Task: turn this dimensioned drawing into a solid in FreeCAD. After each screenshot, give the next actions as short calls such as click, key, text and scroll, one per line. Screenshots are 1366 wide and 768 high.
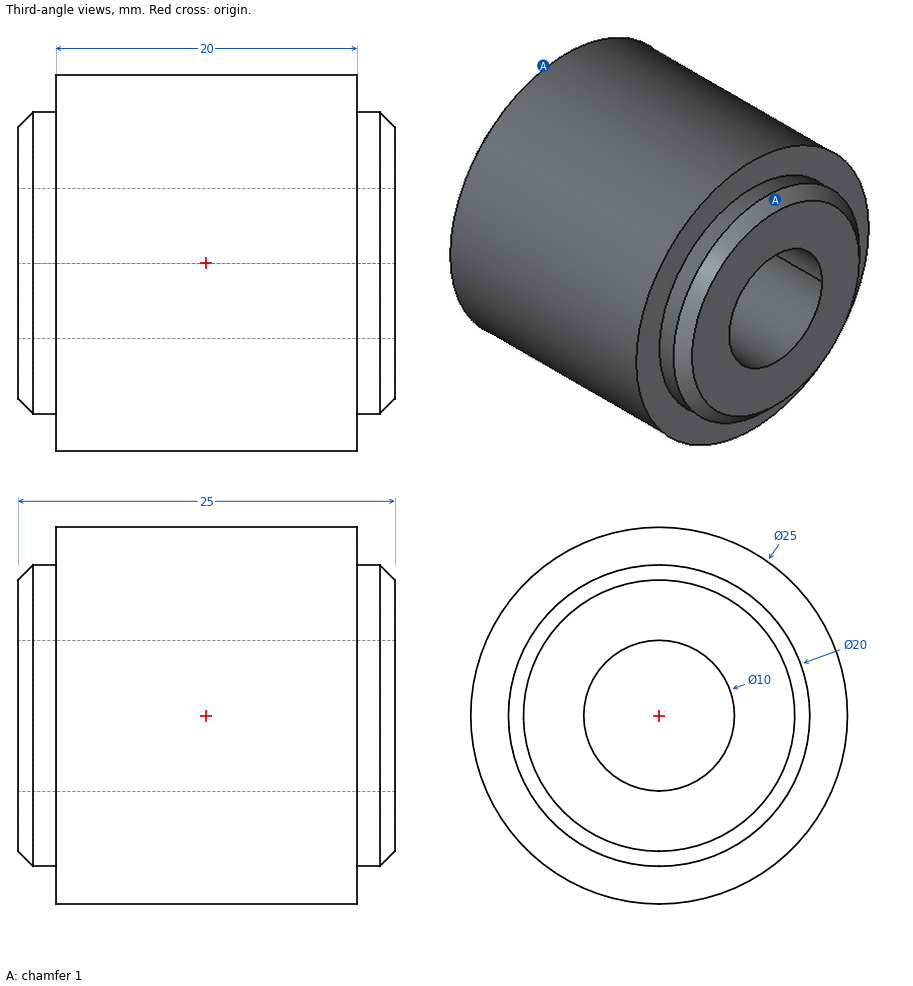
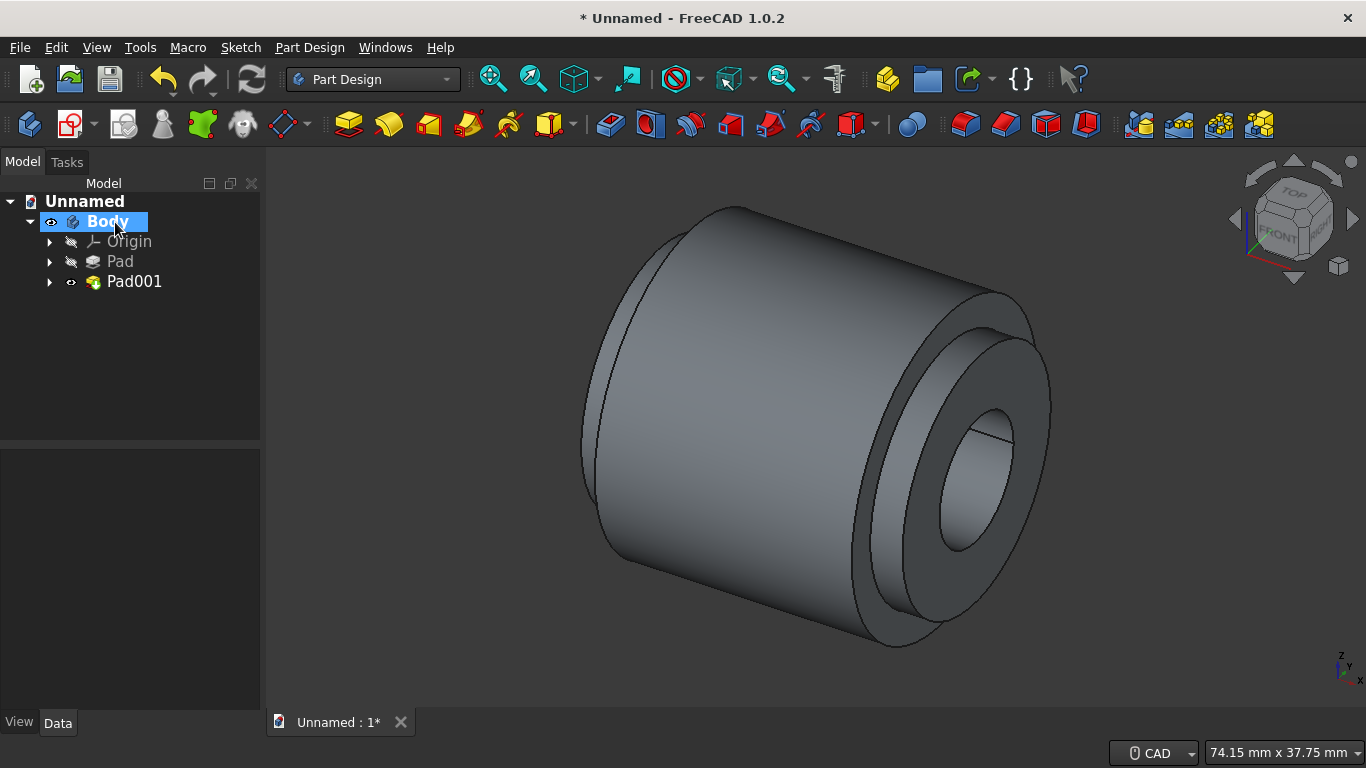
key(v)
key(f)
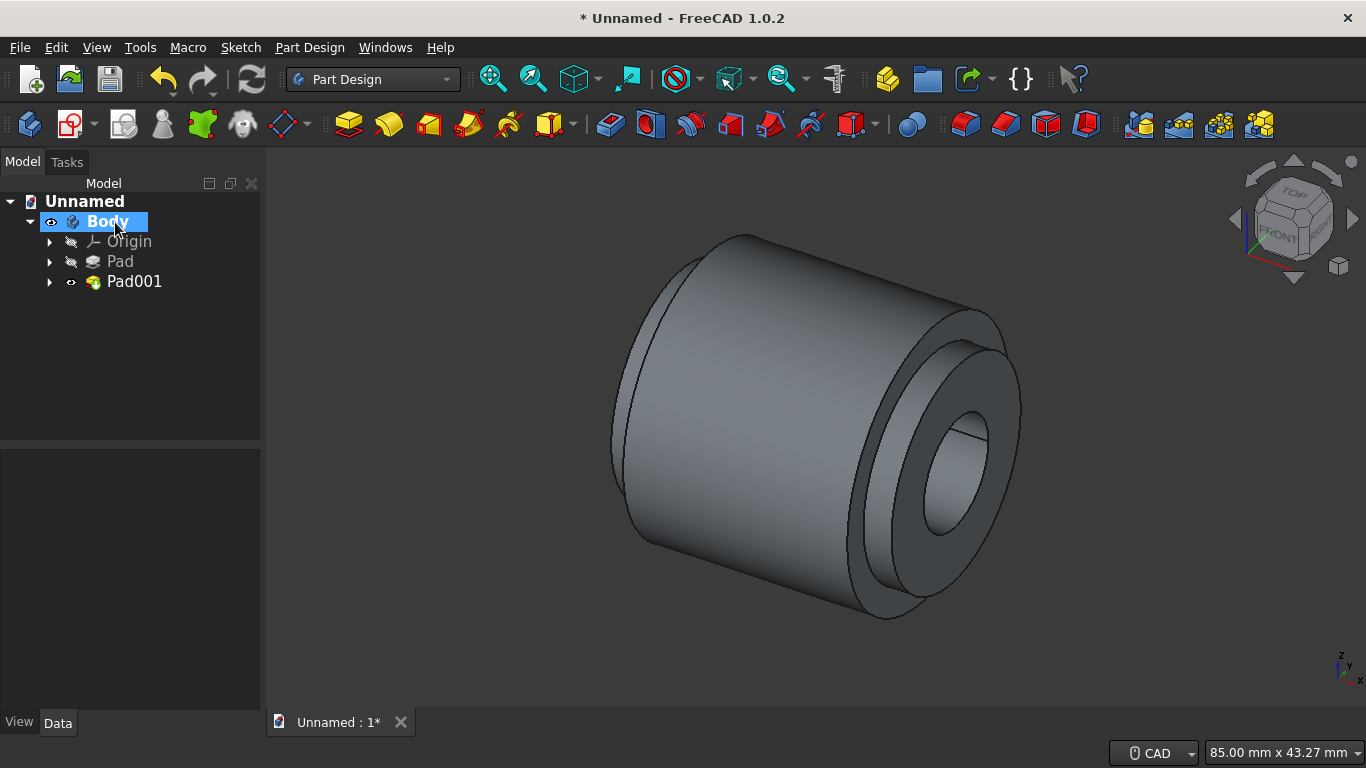
click(891, 537)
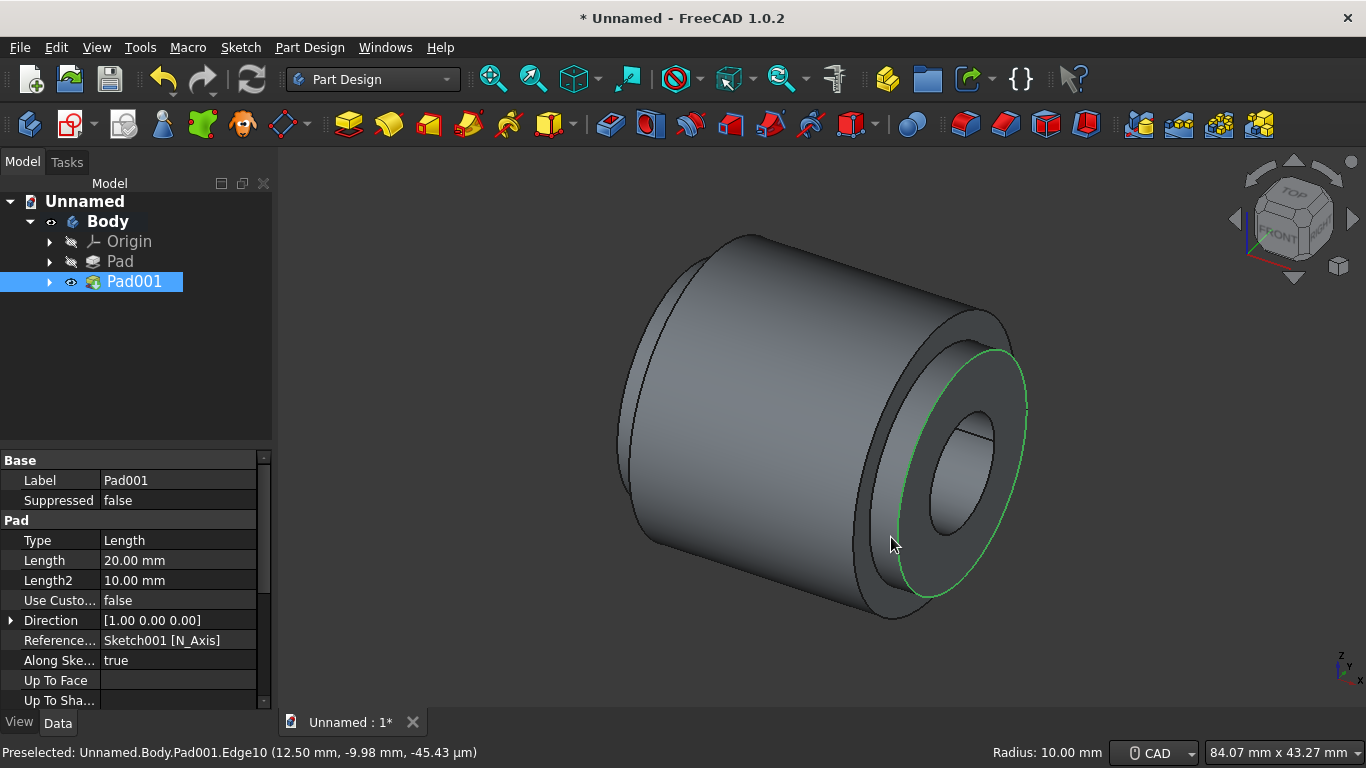
key(0)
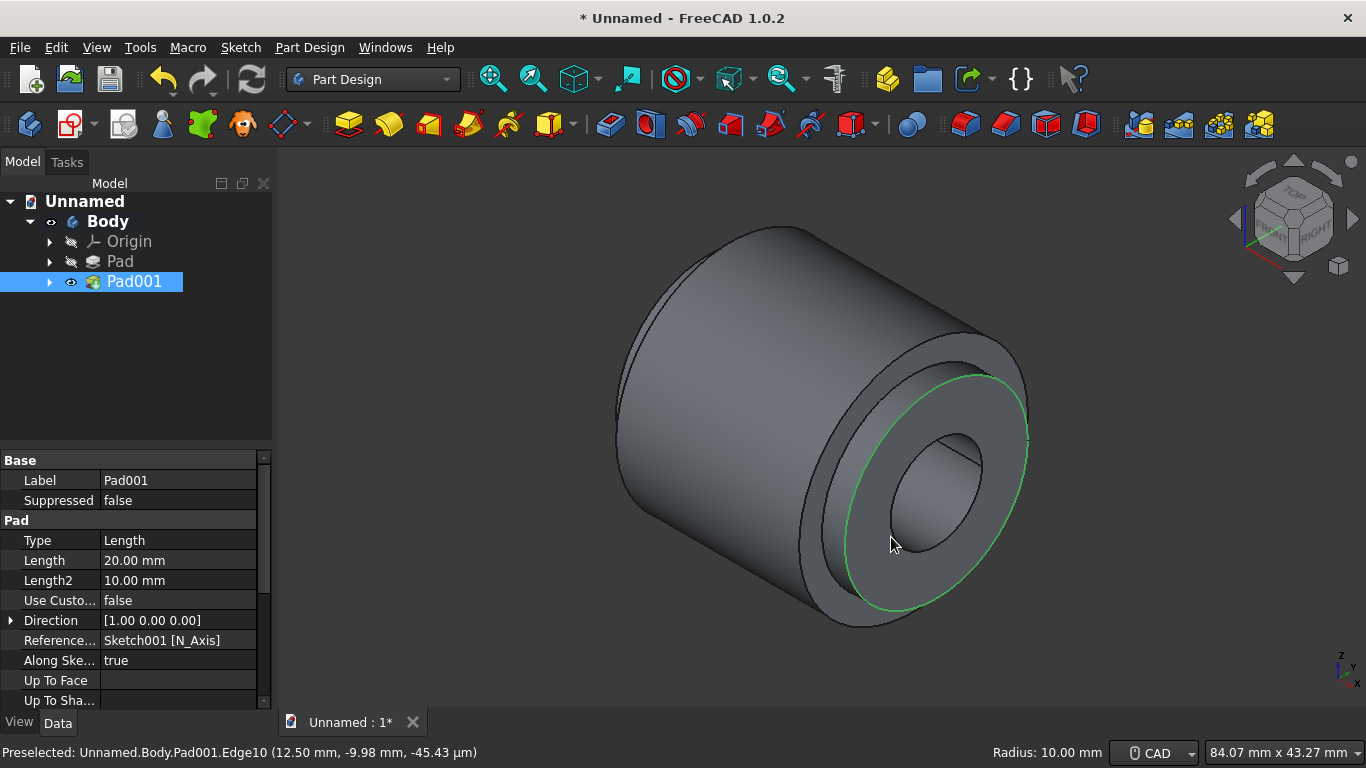
key(2)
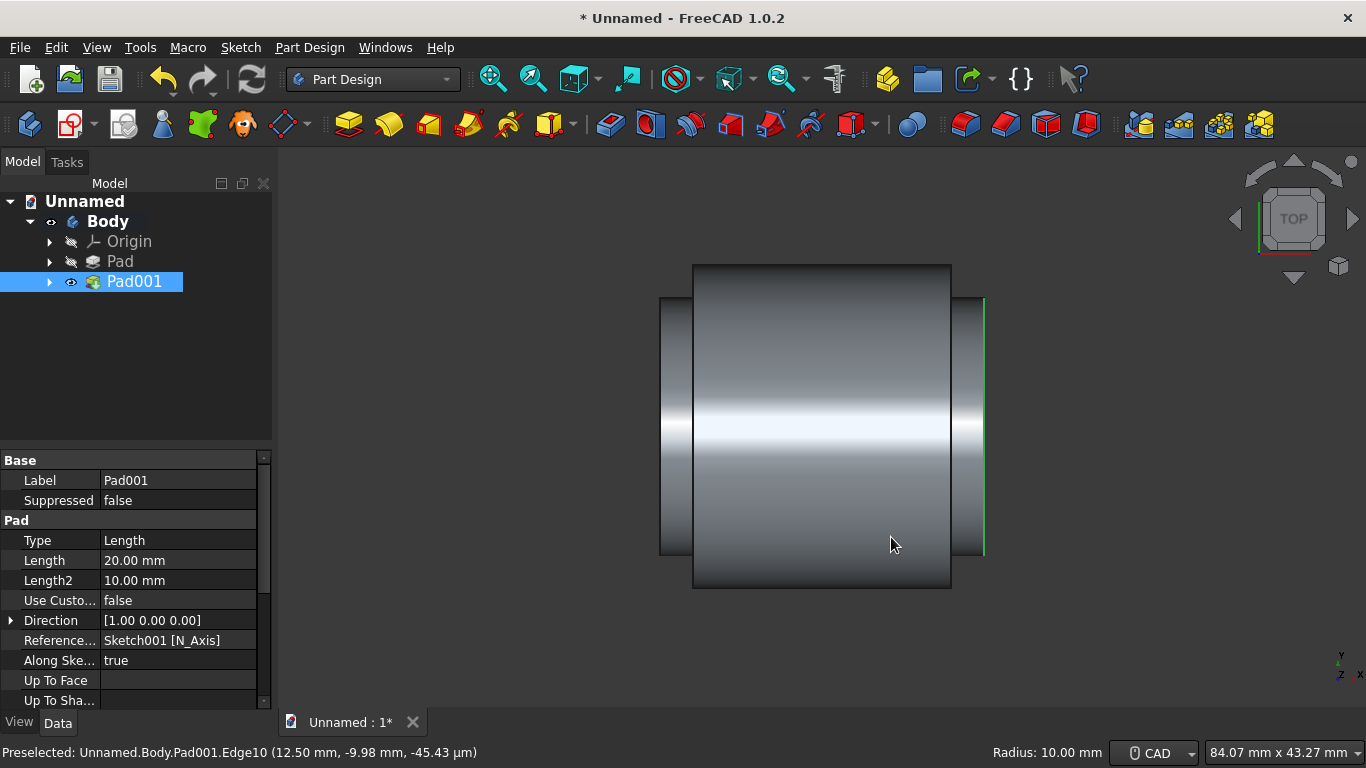
click(660, 531, ctrl)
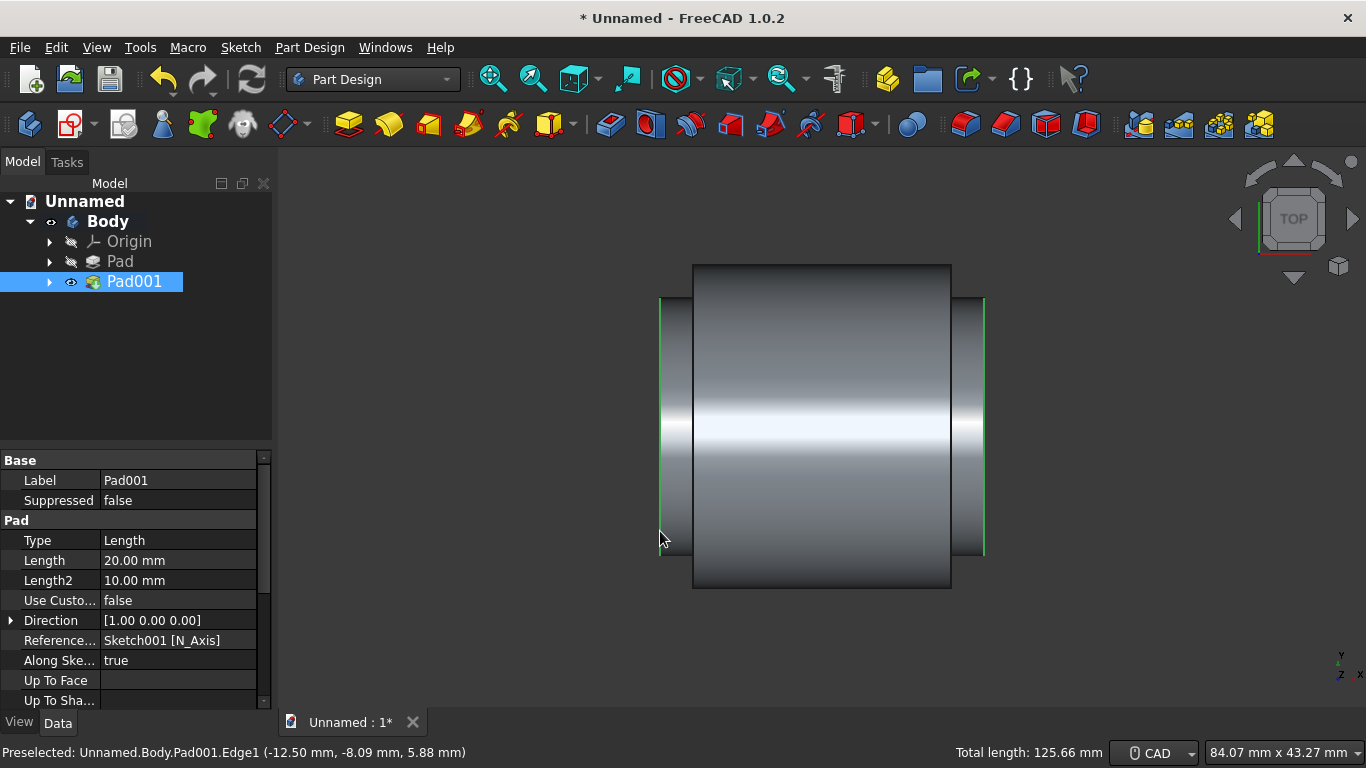
click(1006, 124)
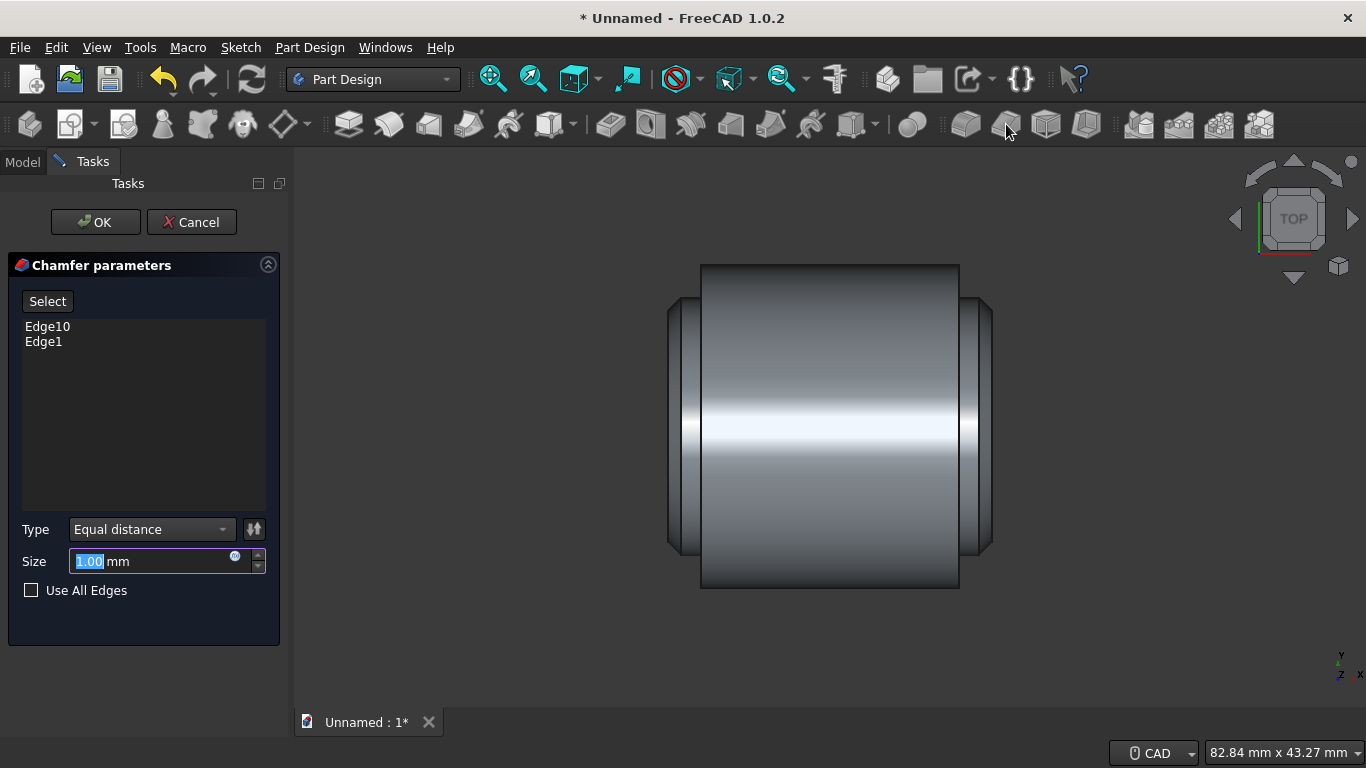
text(1)
key(Tab)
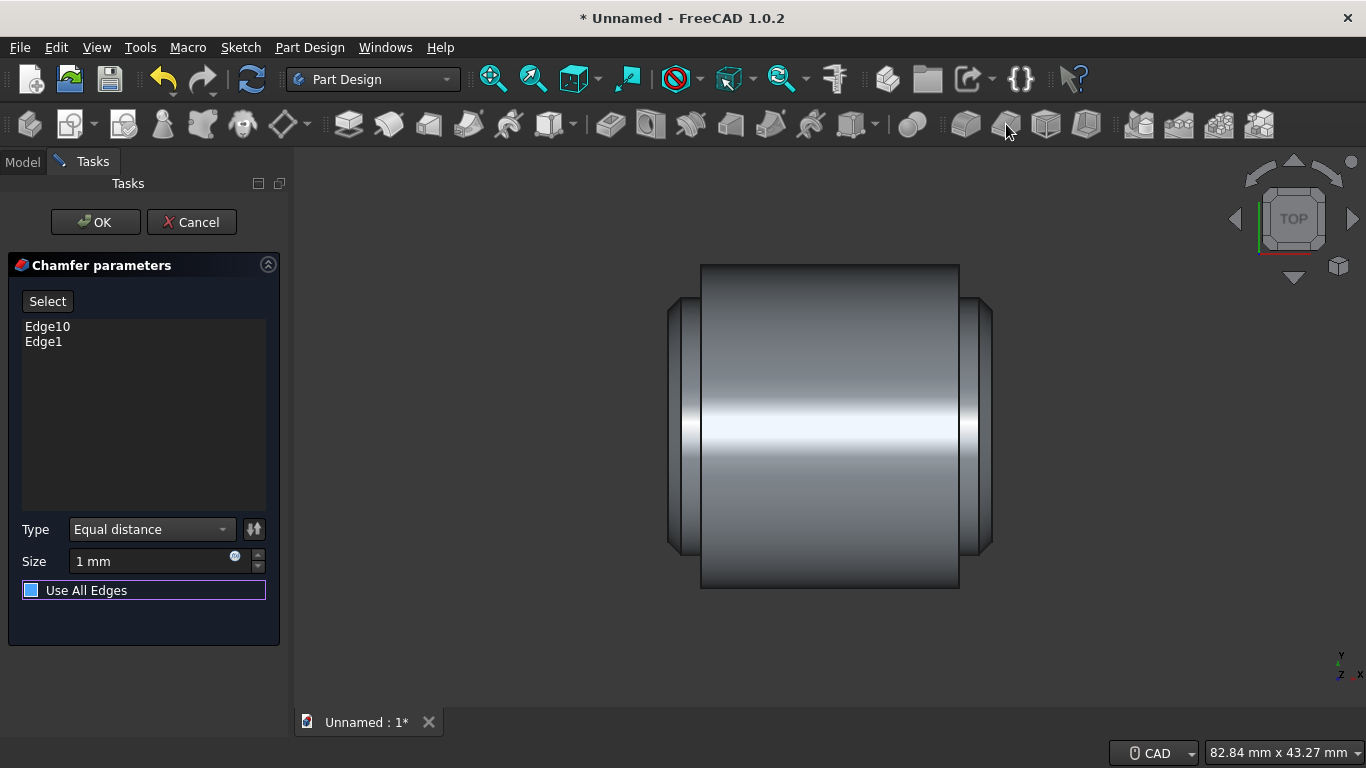
click(96, 222)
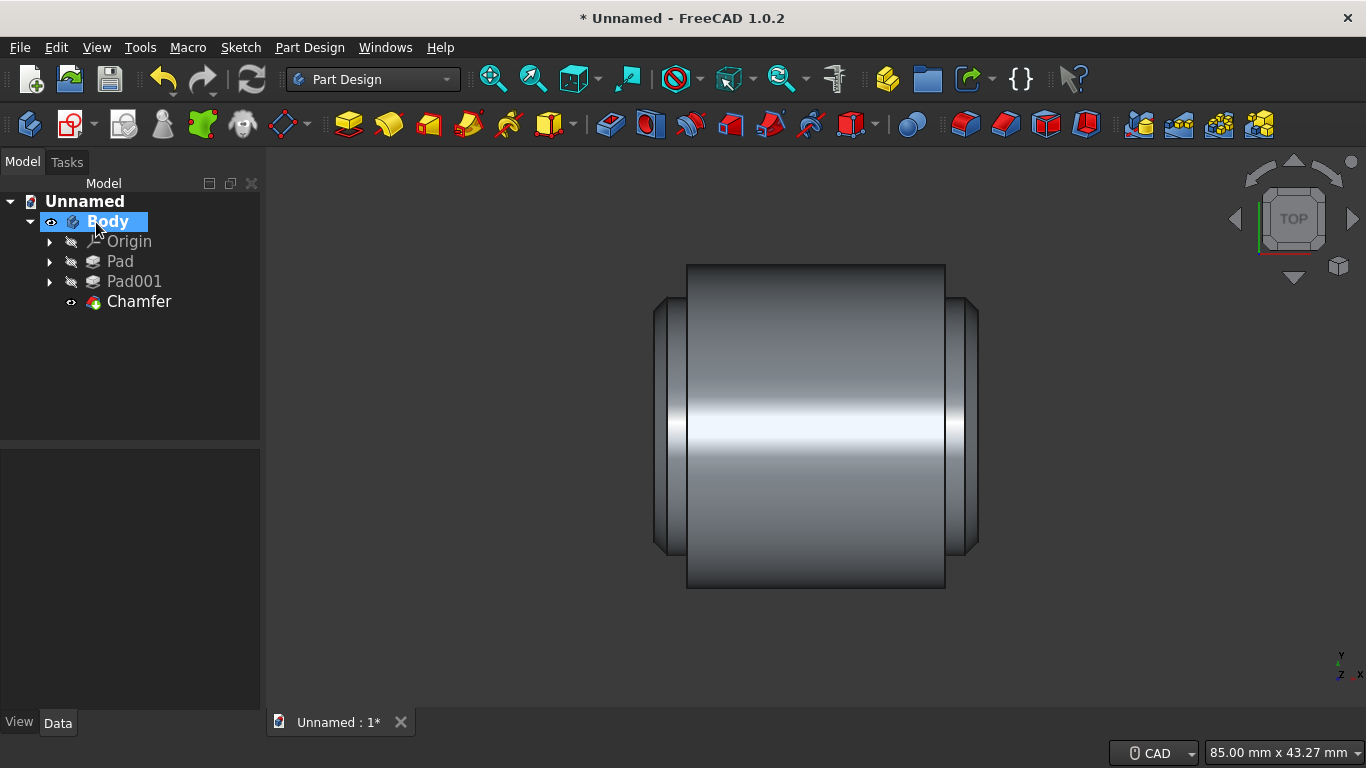
key(0)